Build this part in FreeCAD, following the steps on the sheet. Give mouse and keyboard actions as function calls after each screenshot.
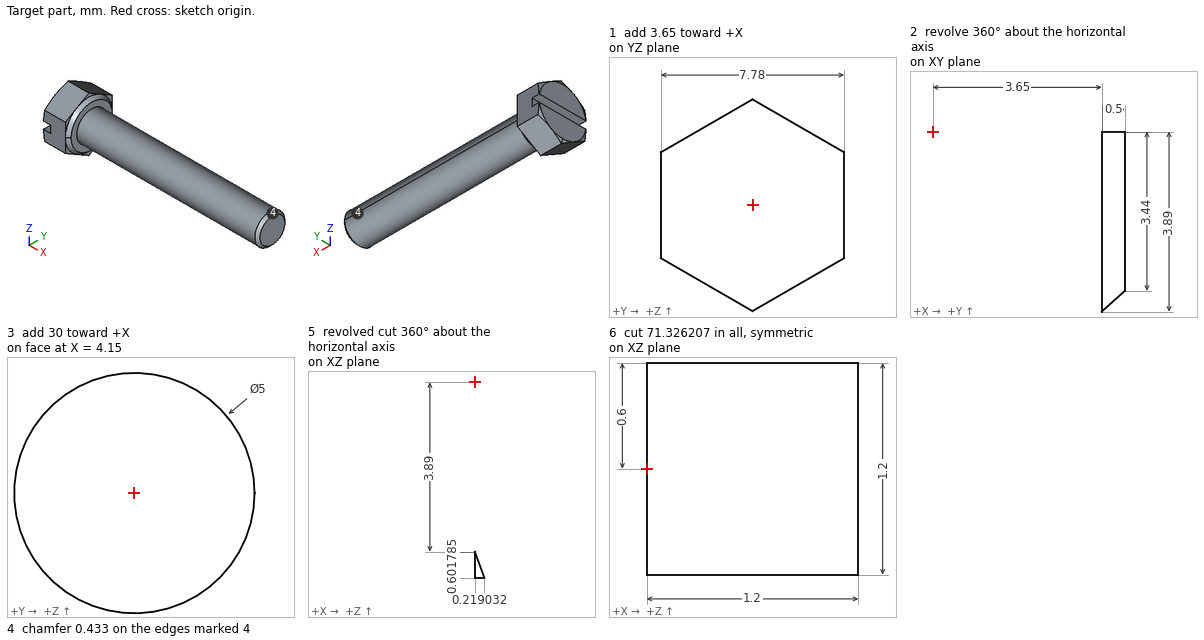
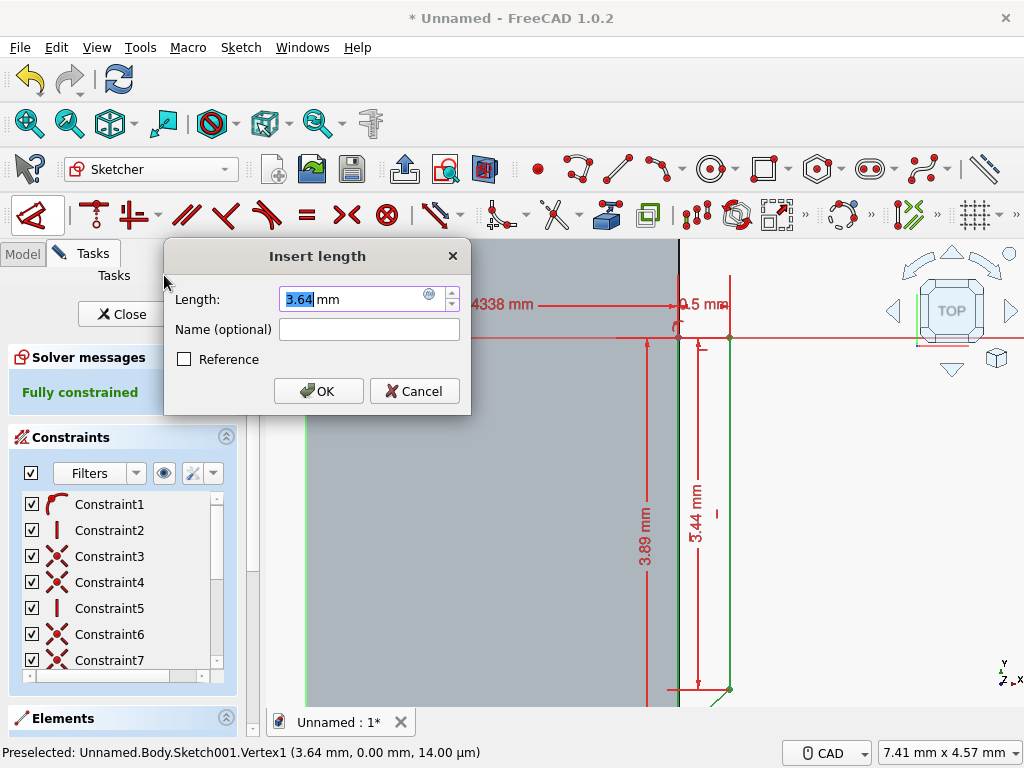
text(3.65)
key(Return)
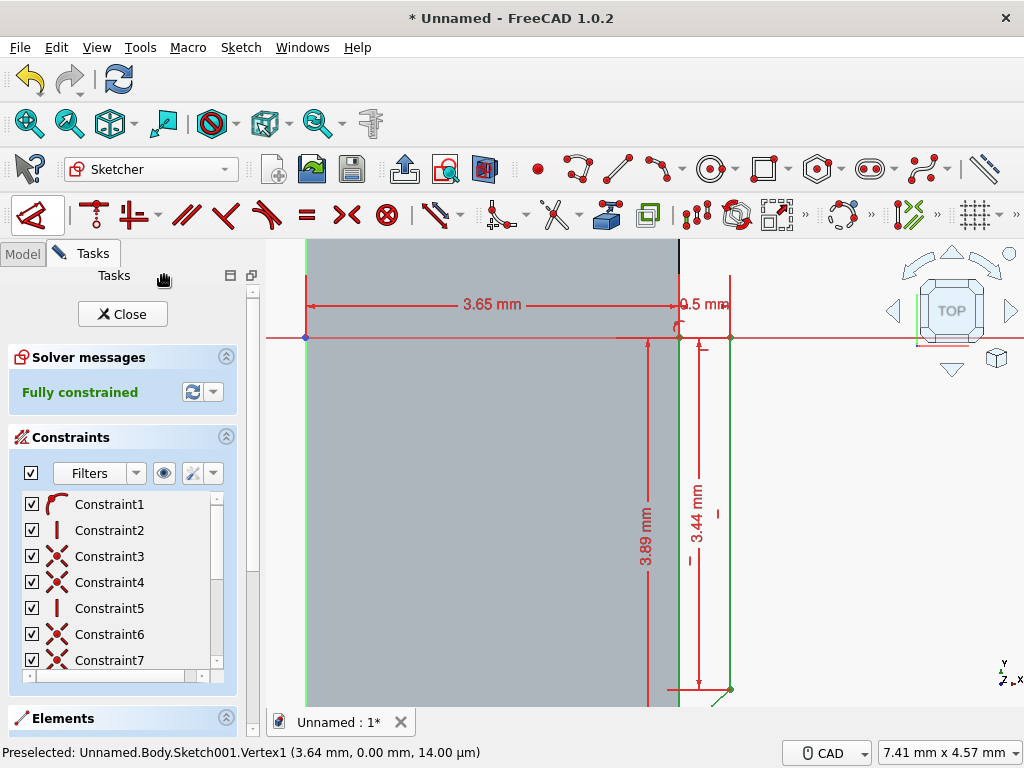
click(123, 314)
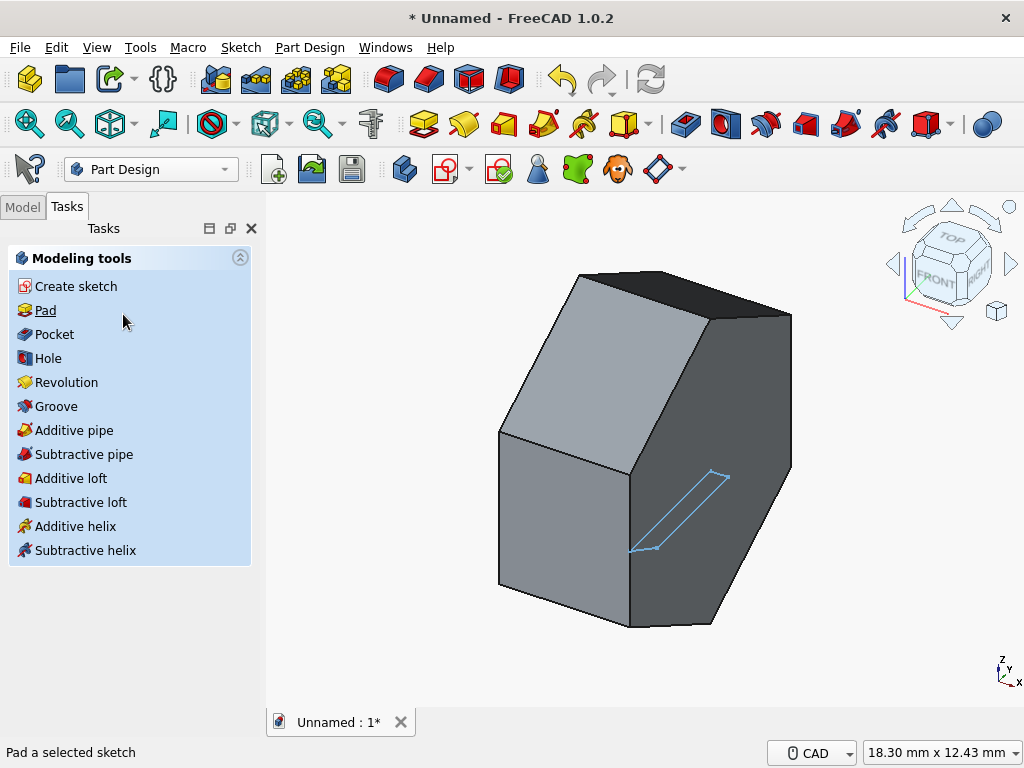
click(464, 124)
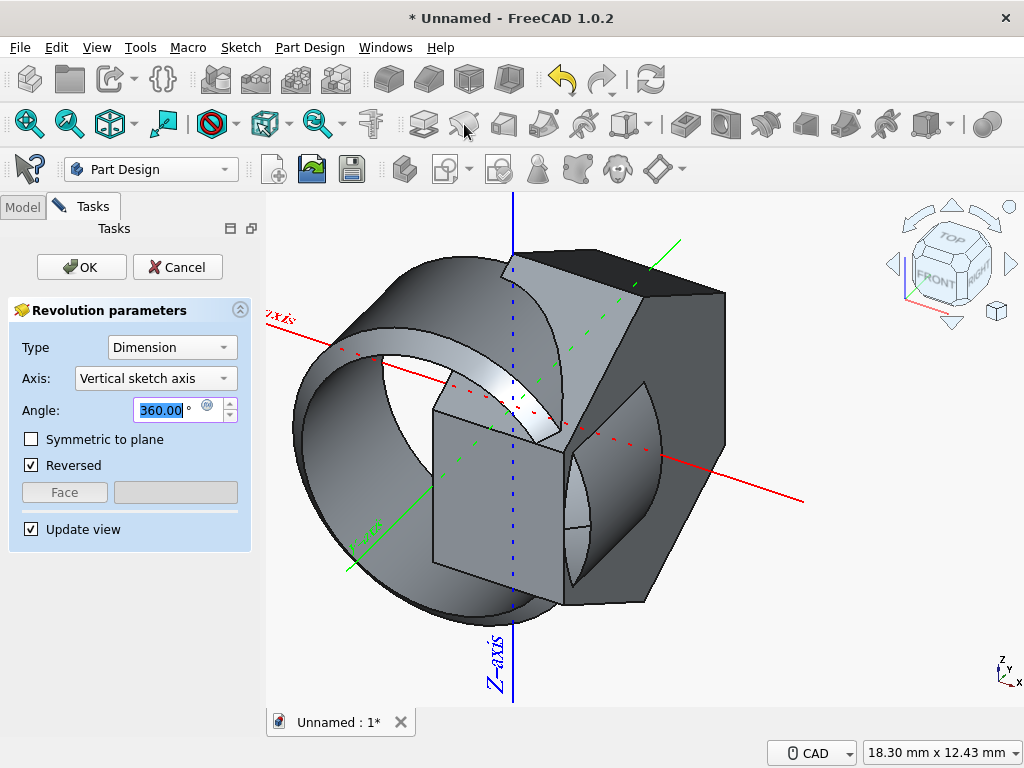
click(156, 378)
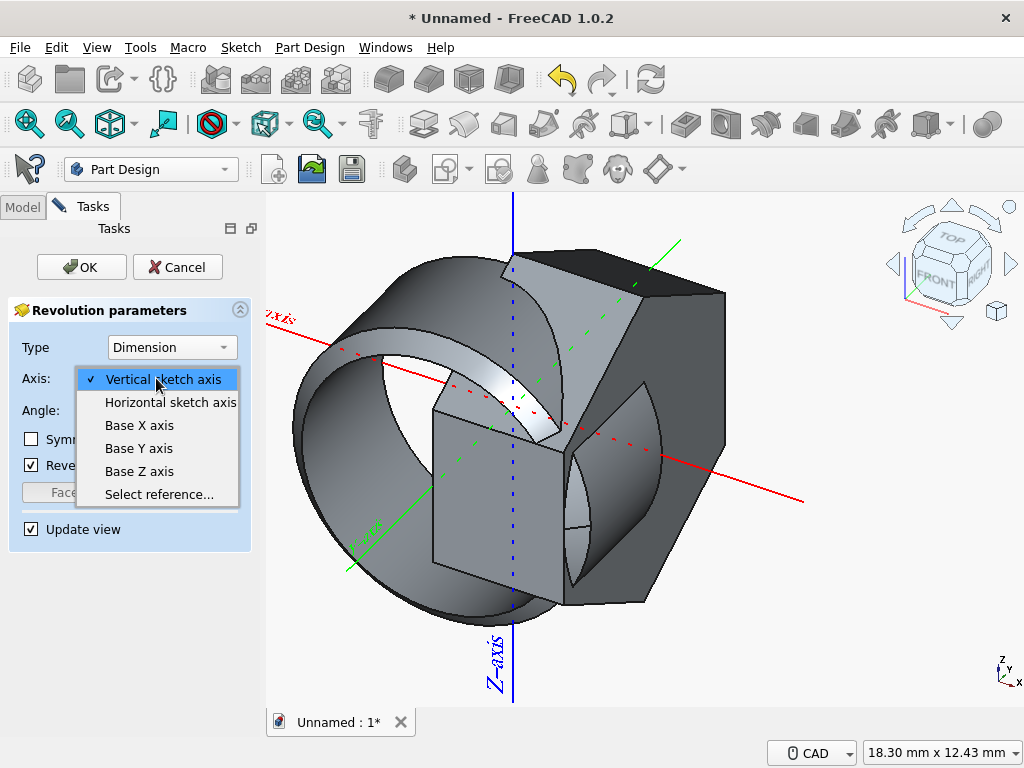
click(156, 402)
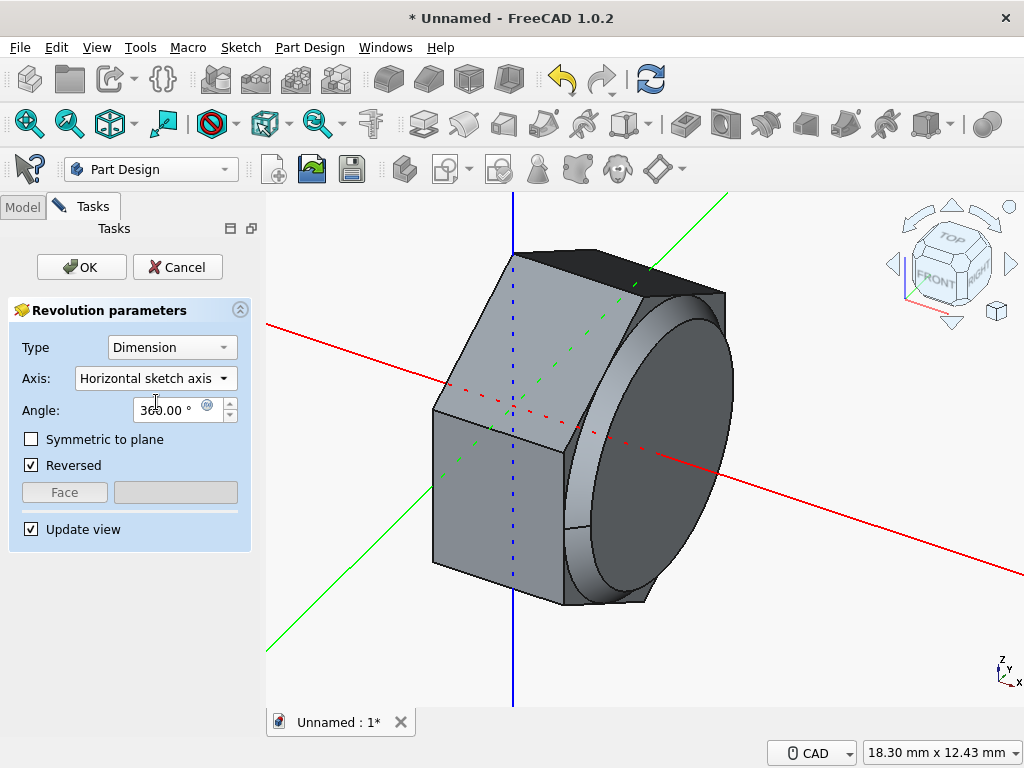
click(82, 267)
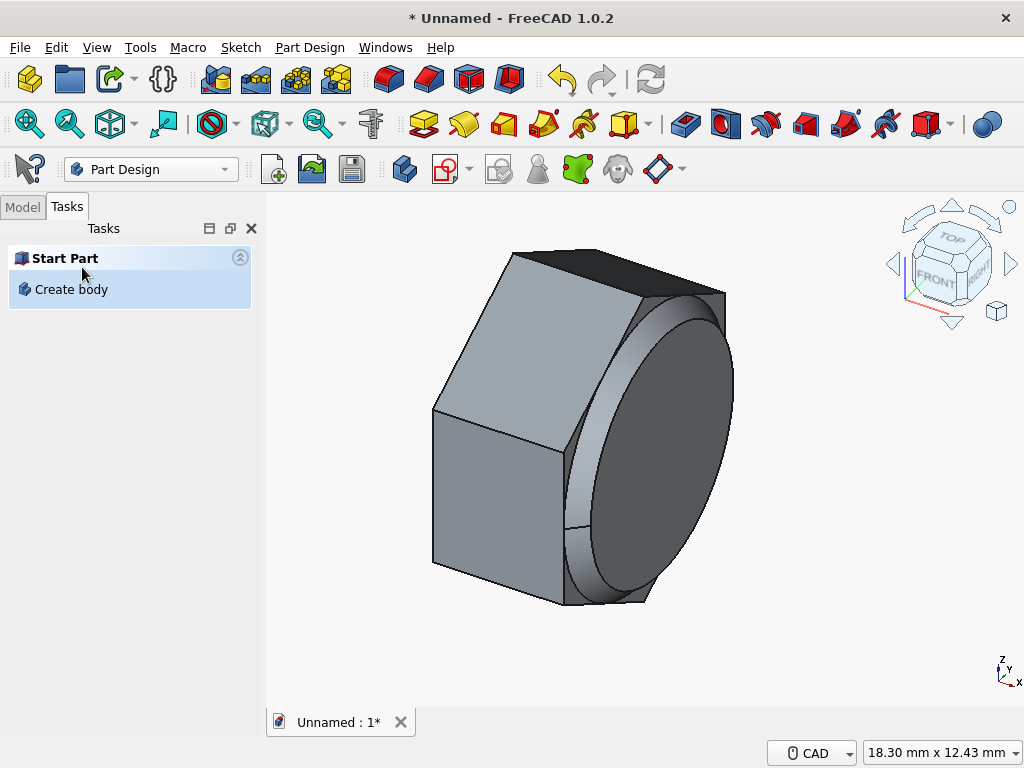
click(30, 124)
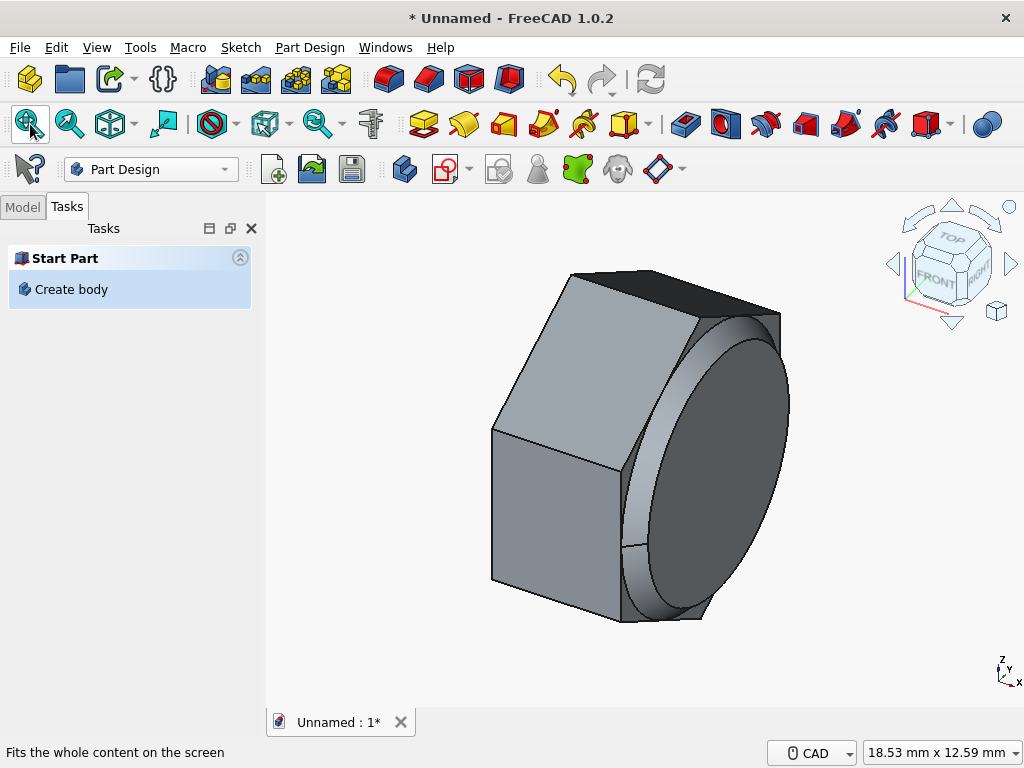
click(719, 473)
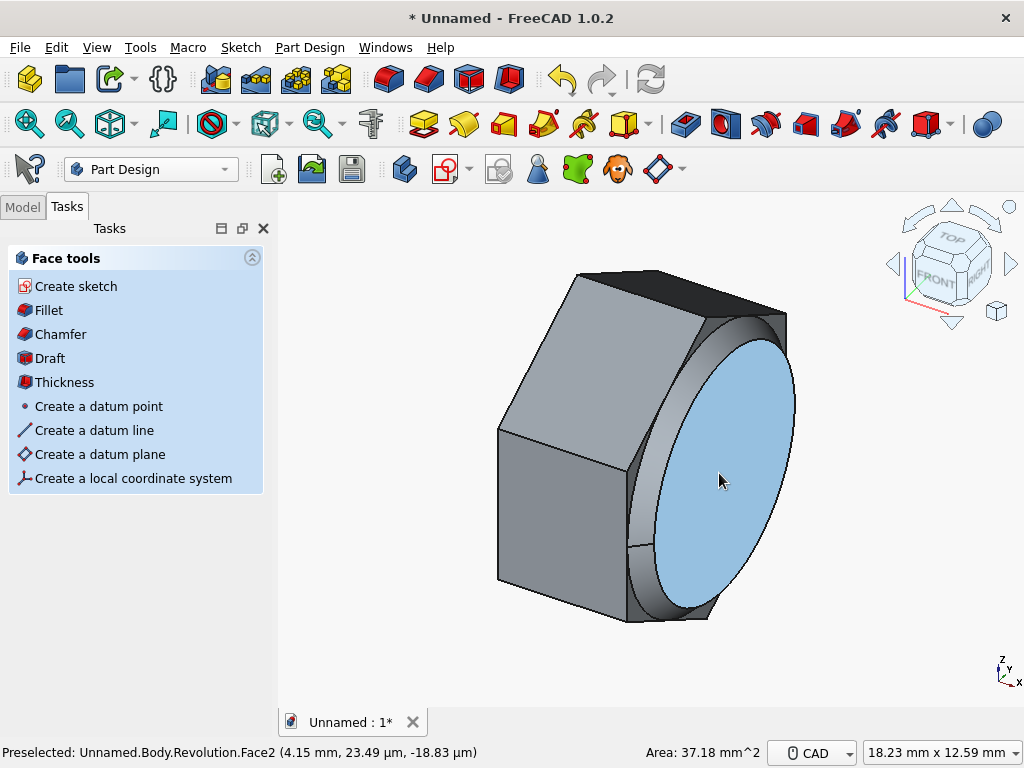
click(446, 170)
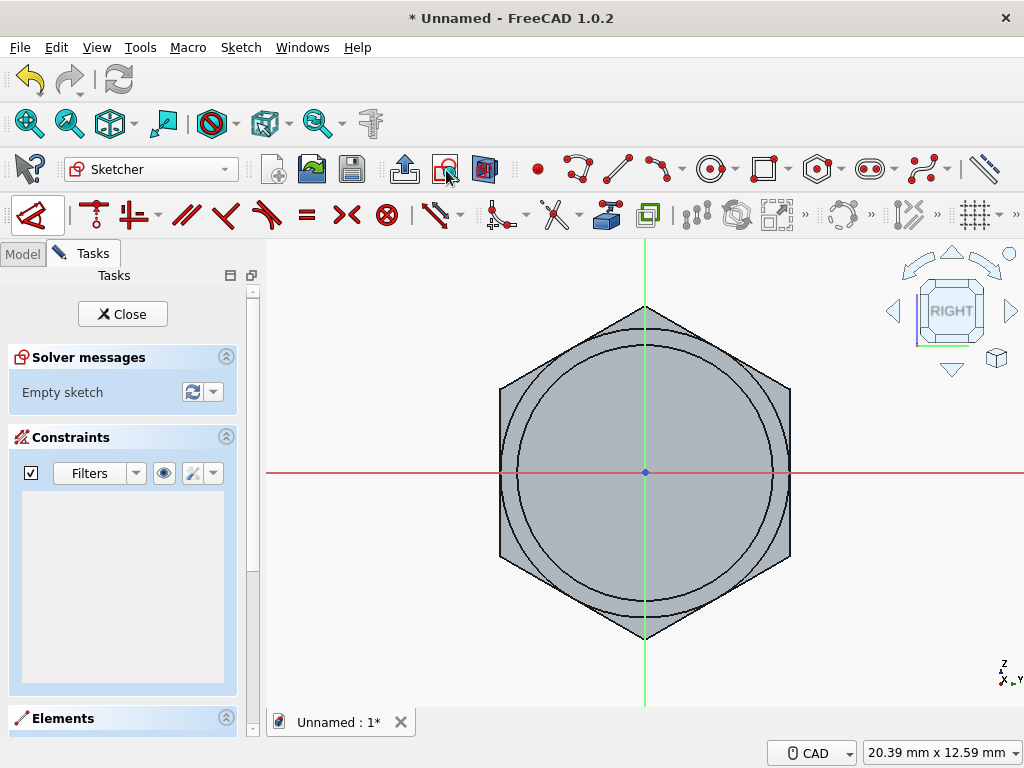
scroll(784, 473, up, 2)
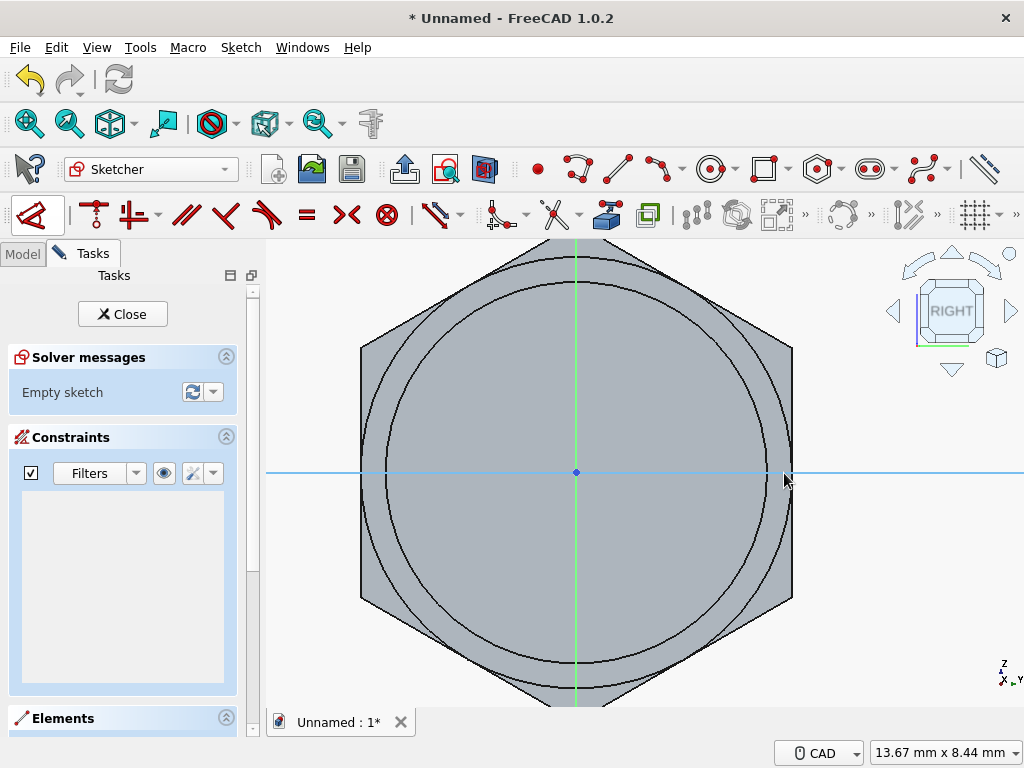
click(712, 170)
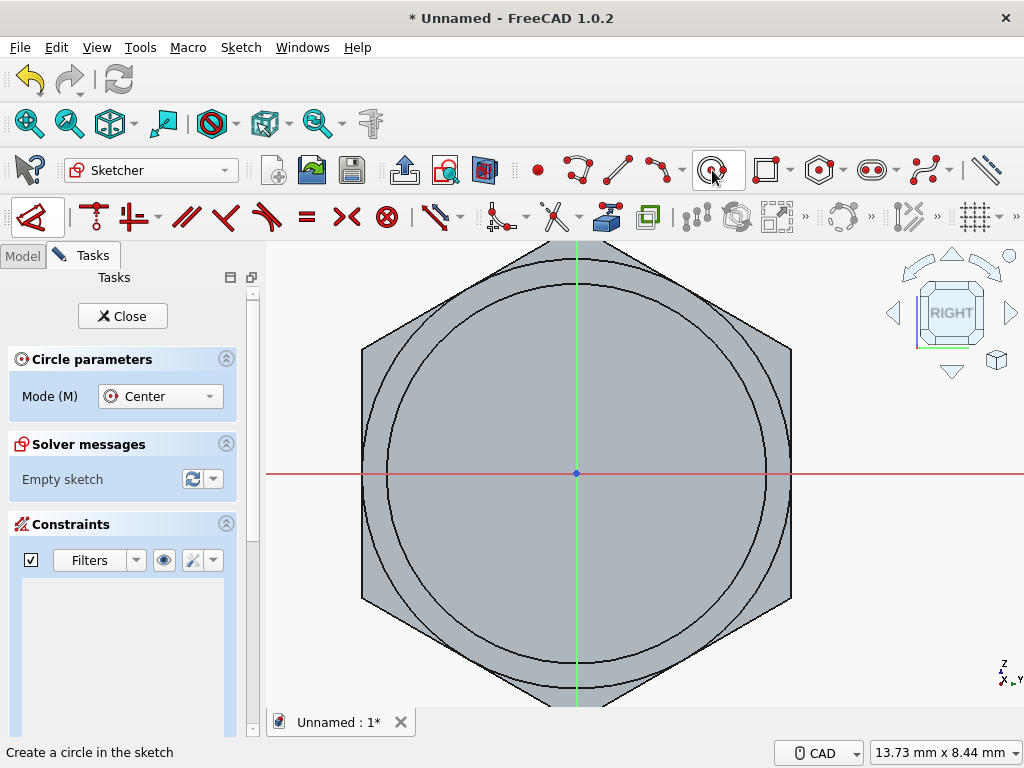
click(577, 474)
move(674, 376)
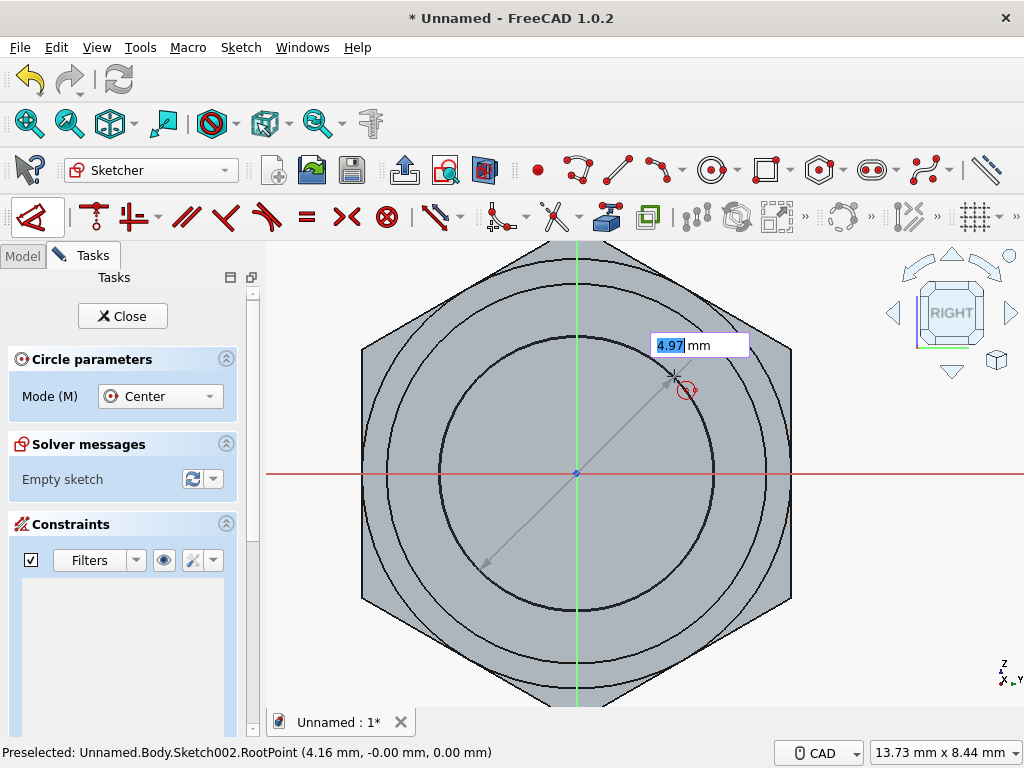
text(5)
key(Return)
key(Escape)